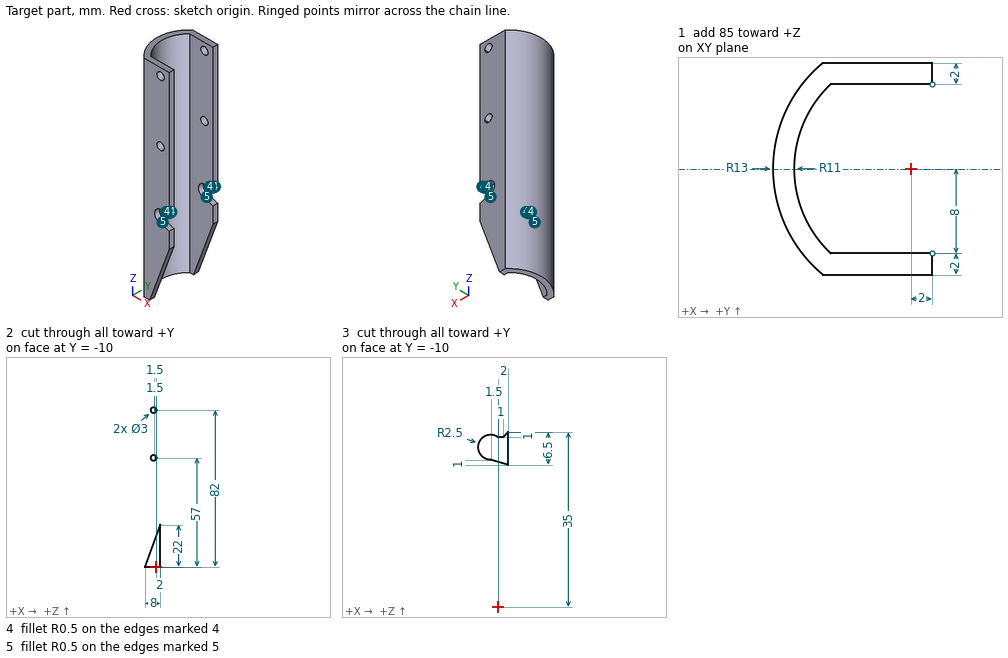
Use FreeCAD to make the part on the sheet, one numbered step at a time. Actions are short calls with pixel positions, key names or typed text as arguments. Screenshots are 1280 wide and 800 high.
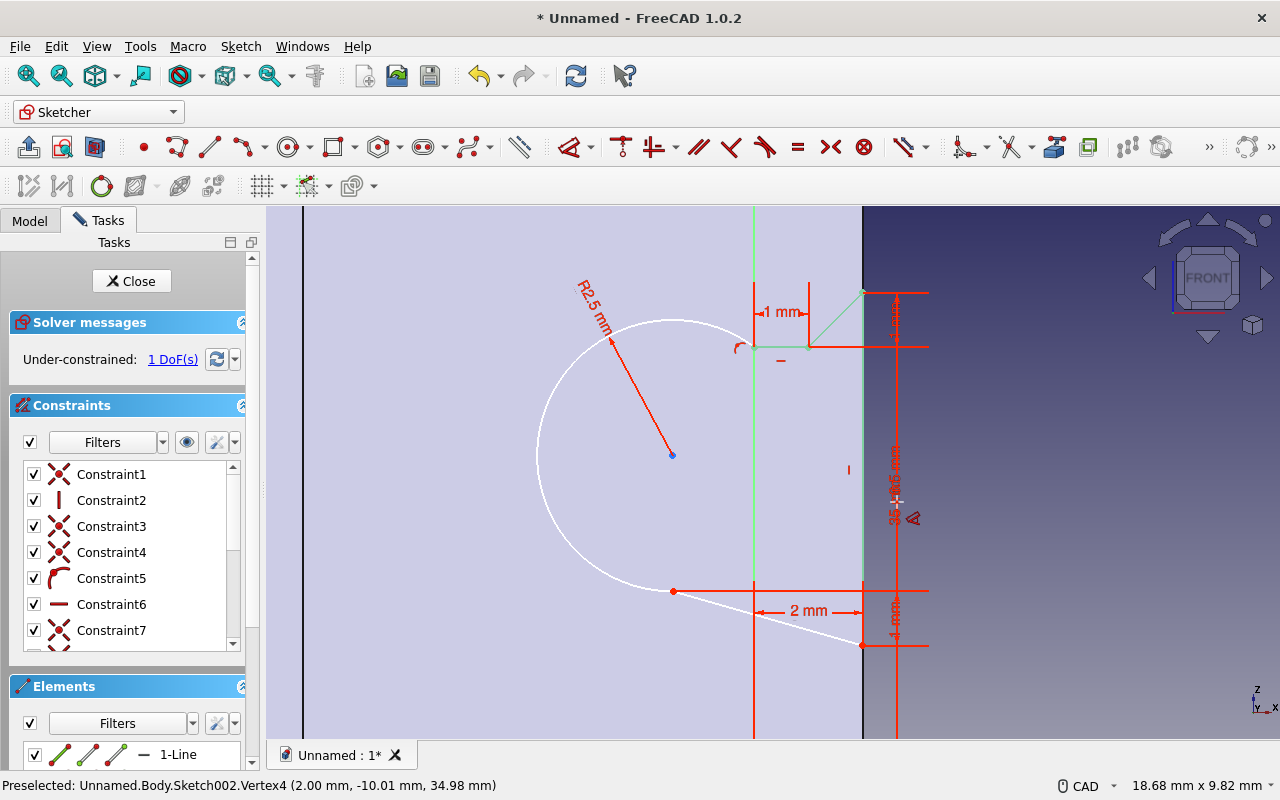
click(673, 591)
click(714, 557)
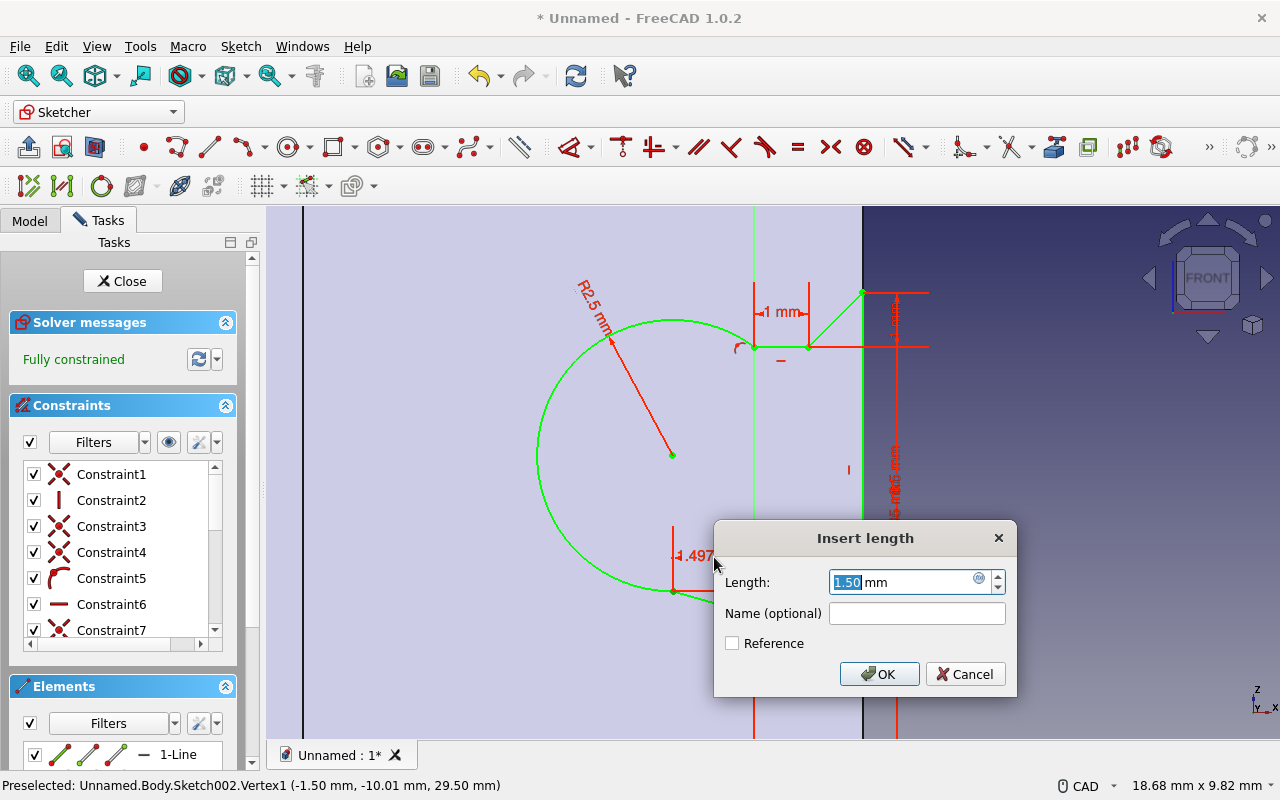
text(1.5)
key(Return)
key(Escape)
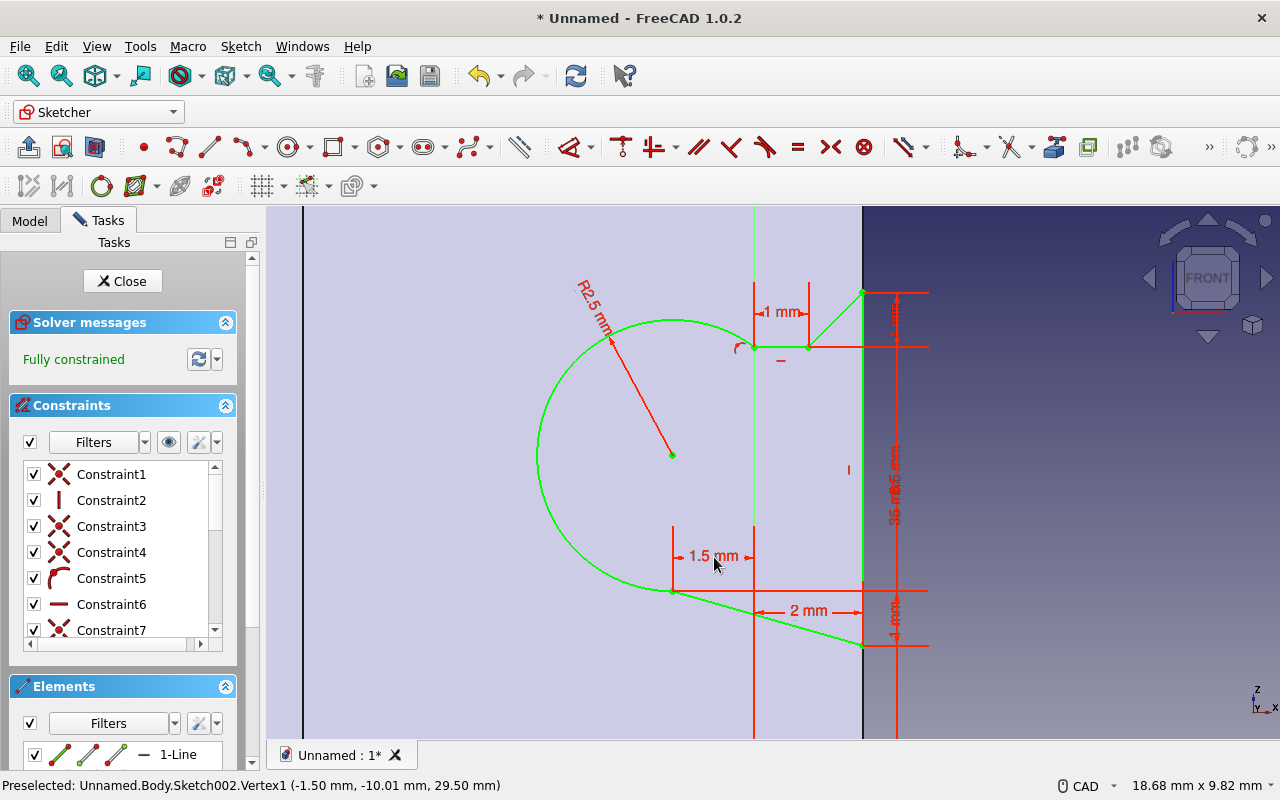
click(123, 281)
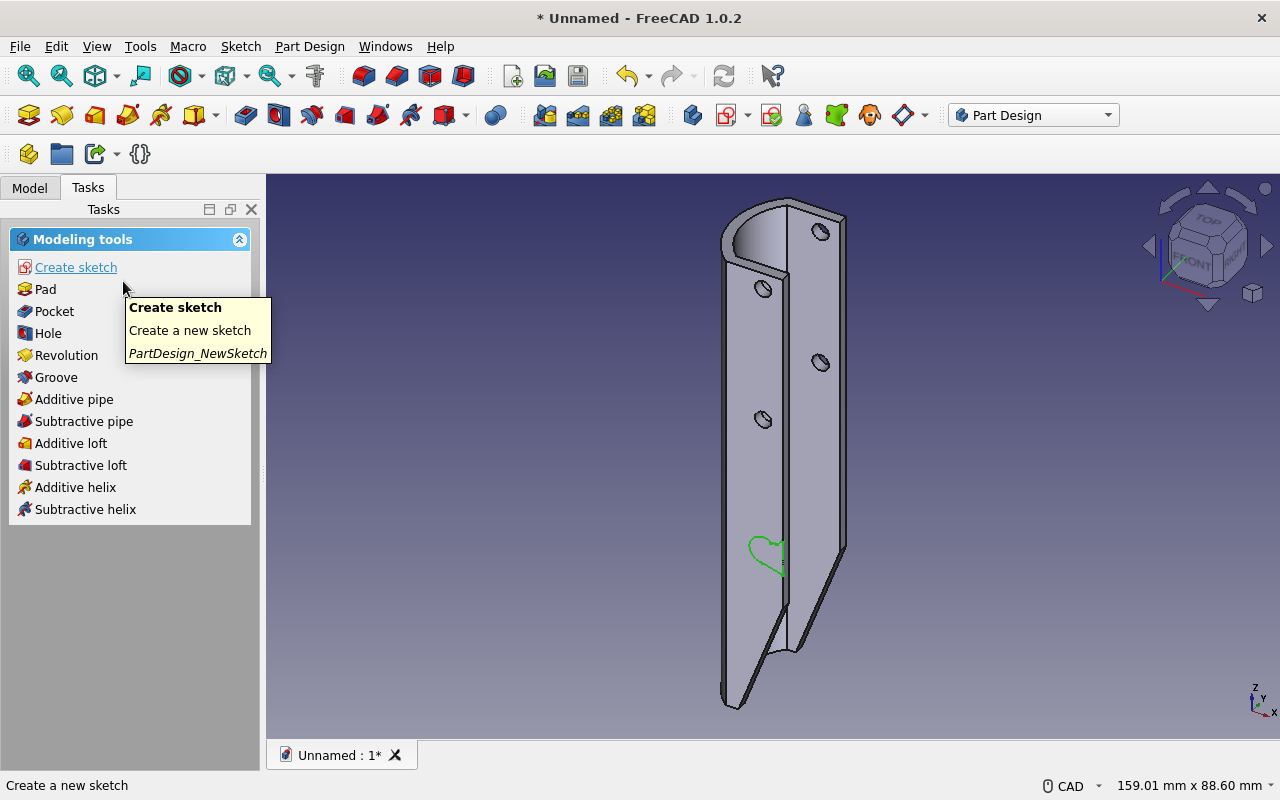
click(246, 116)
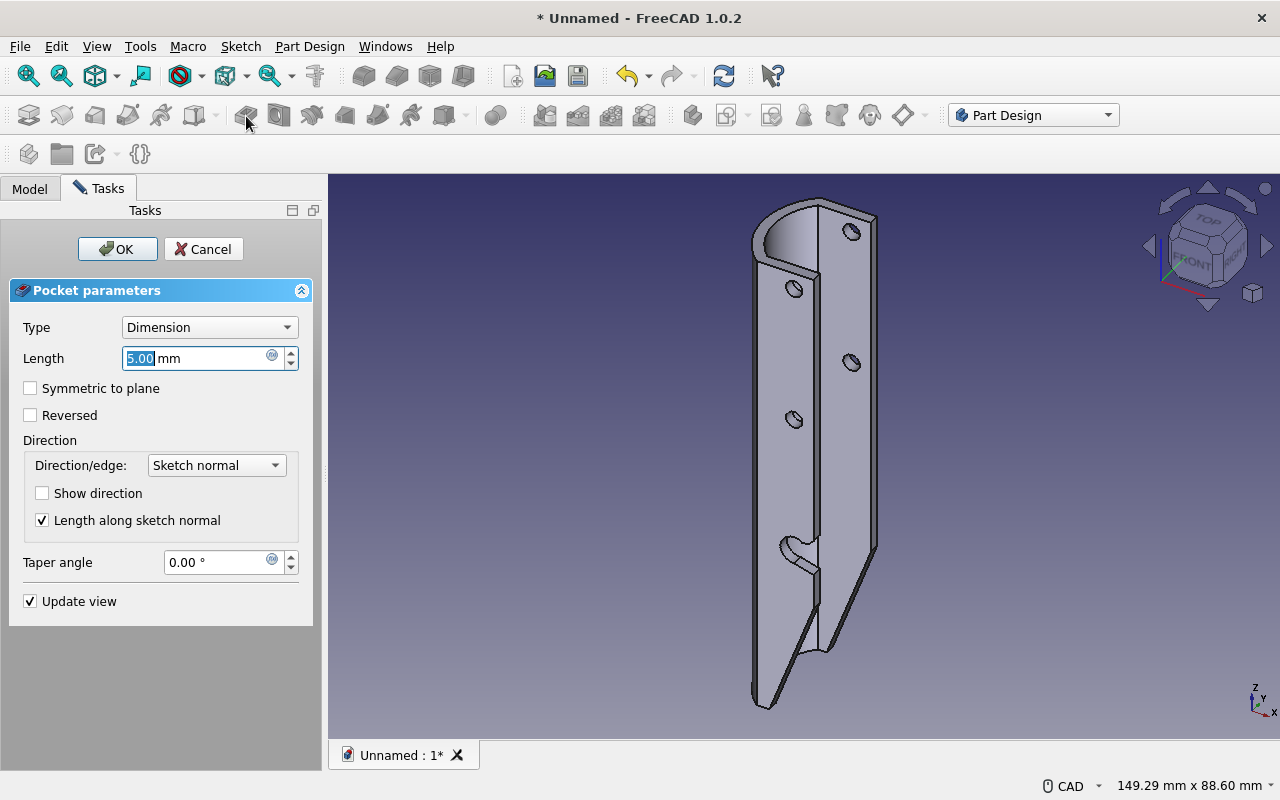
click(210, 328)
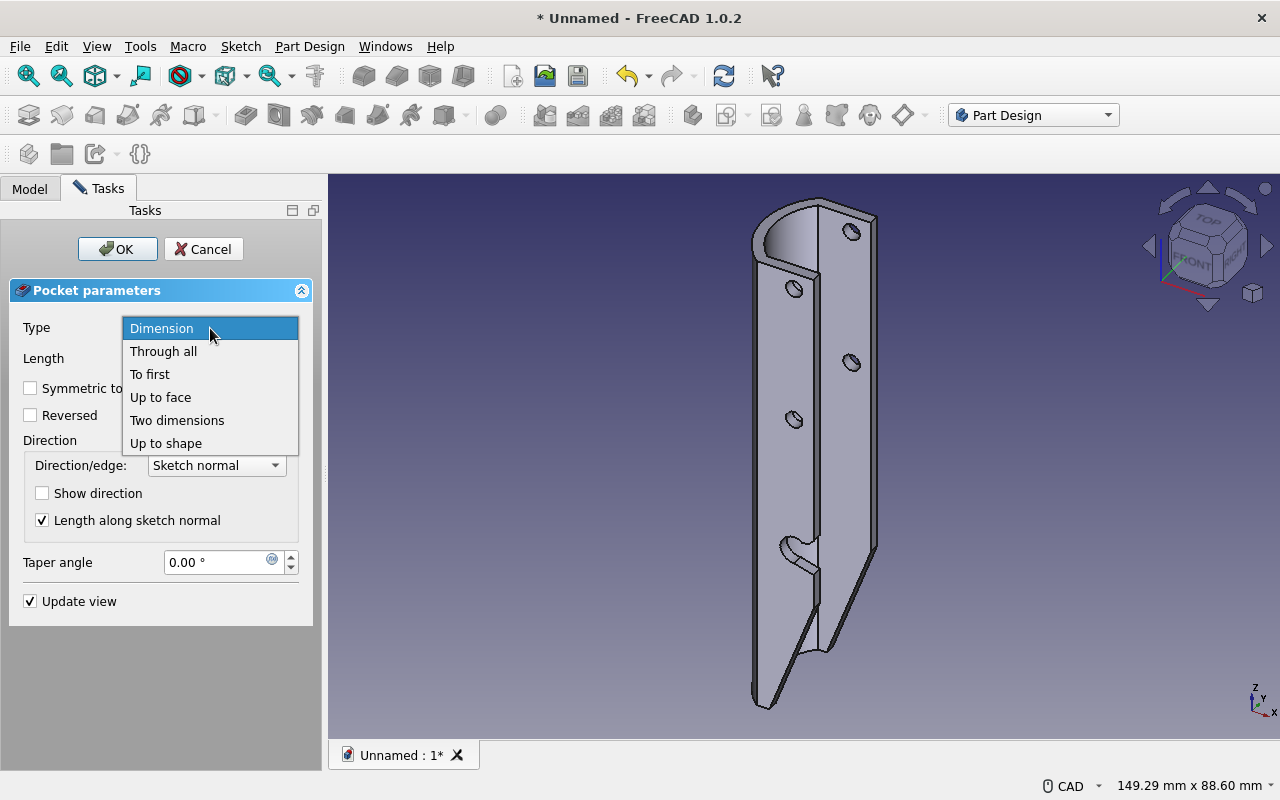
click(208, 352)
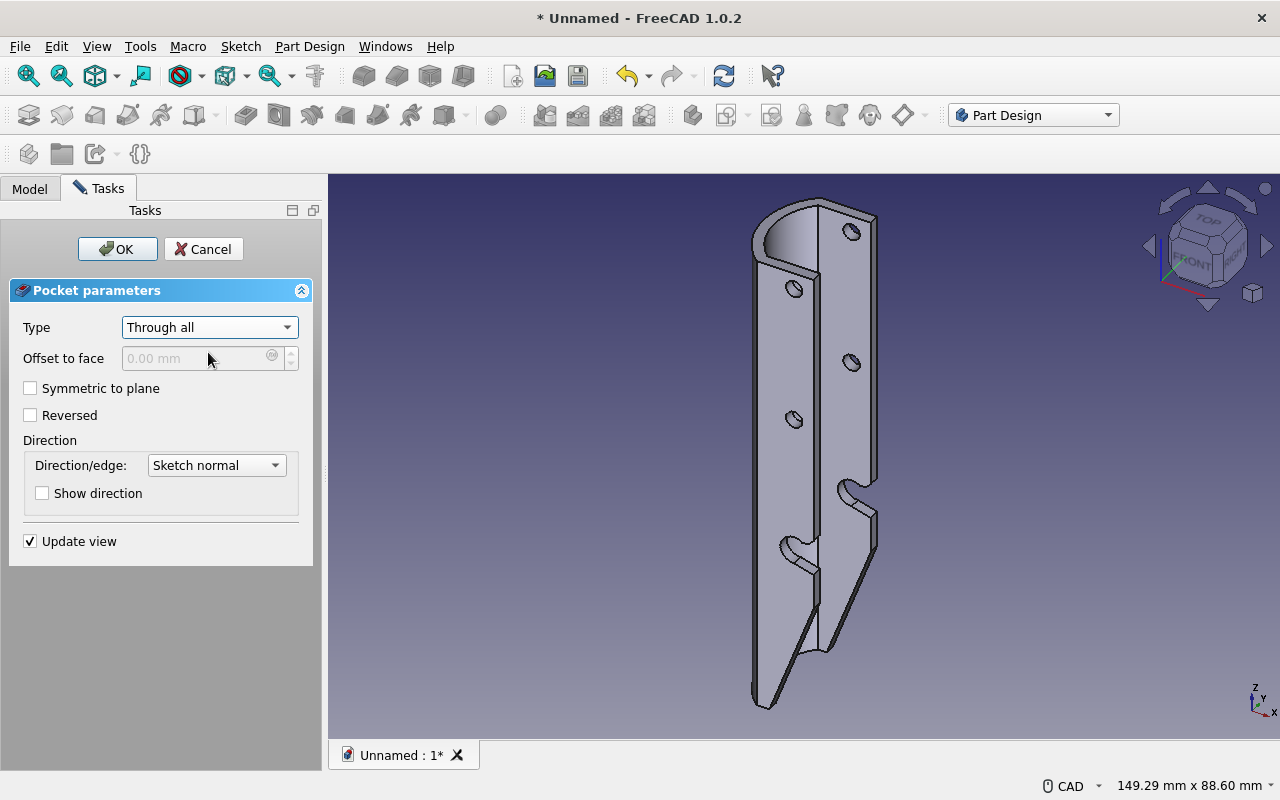
click(118, 249)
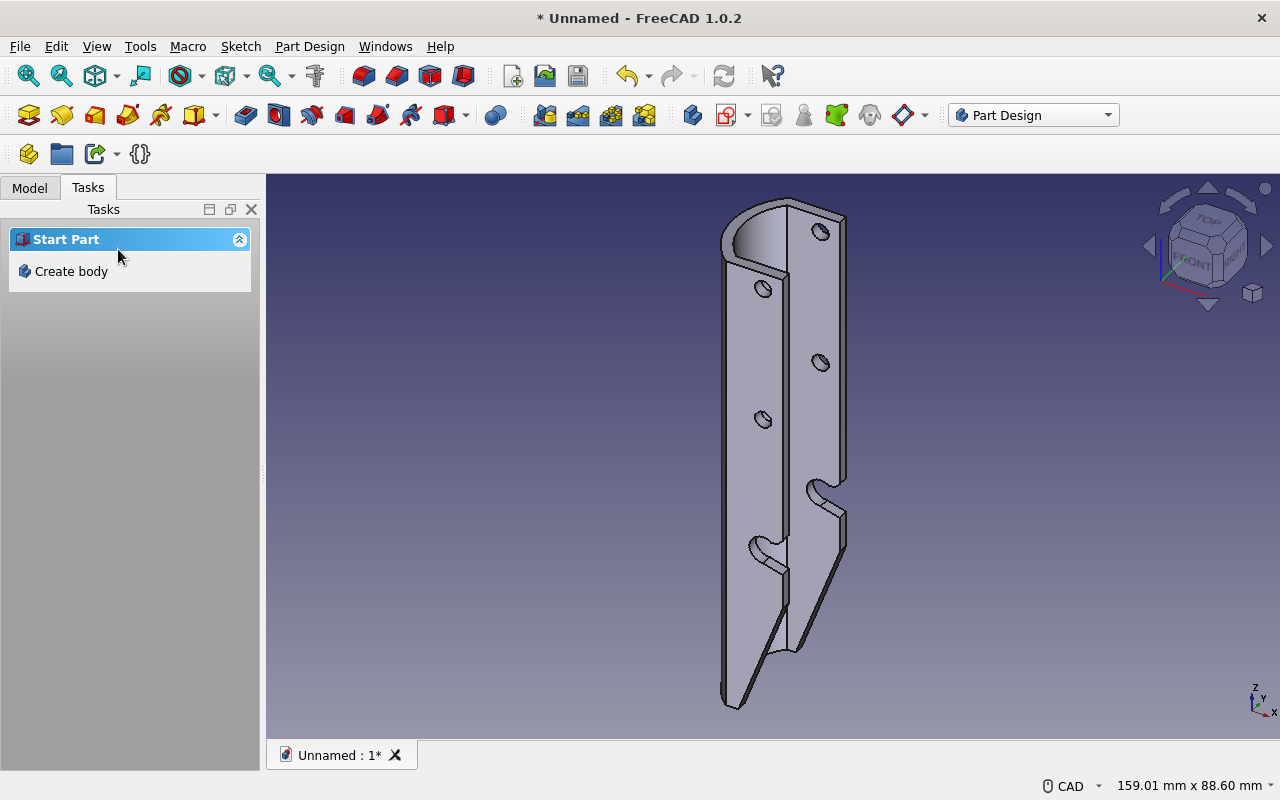
scroll(780, 540, up, 6)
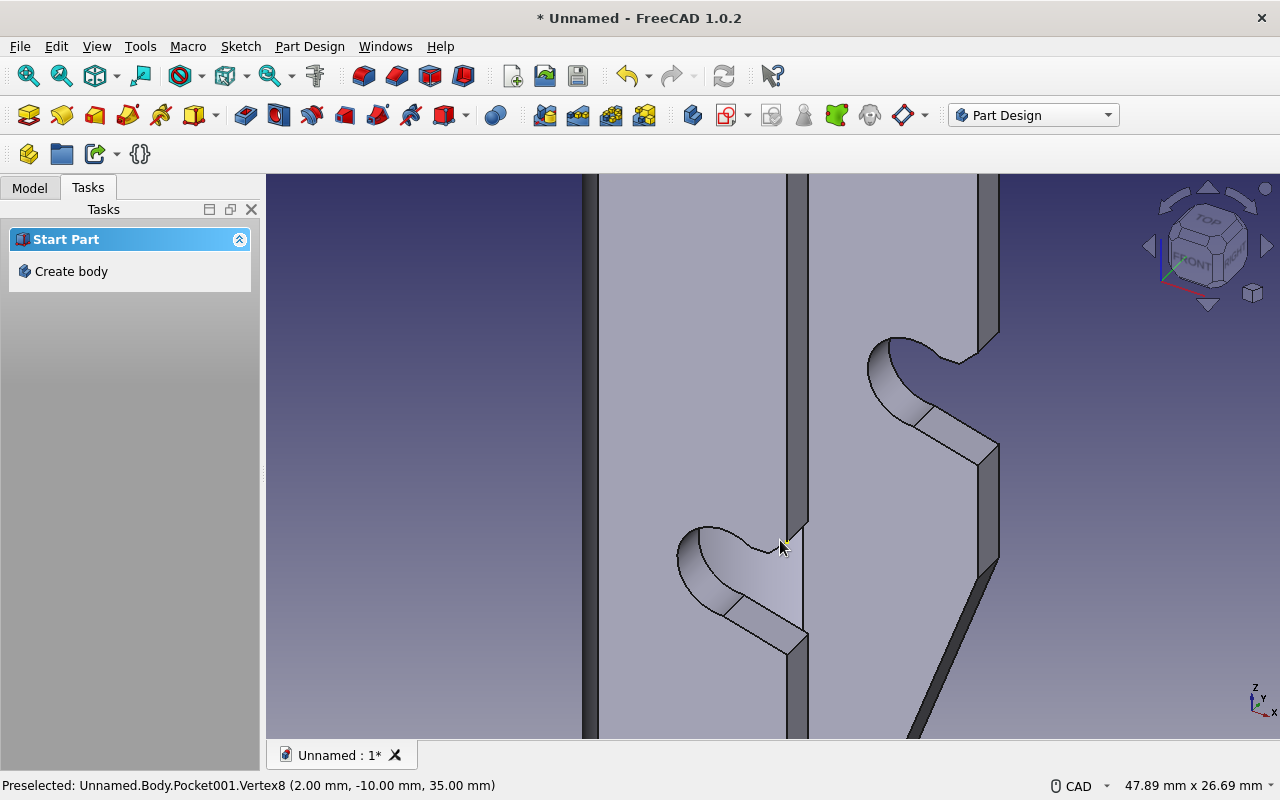
key(v)
key(f)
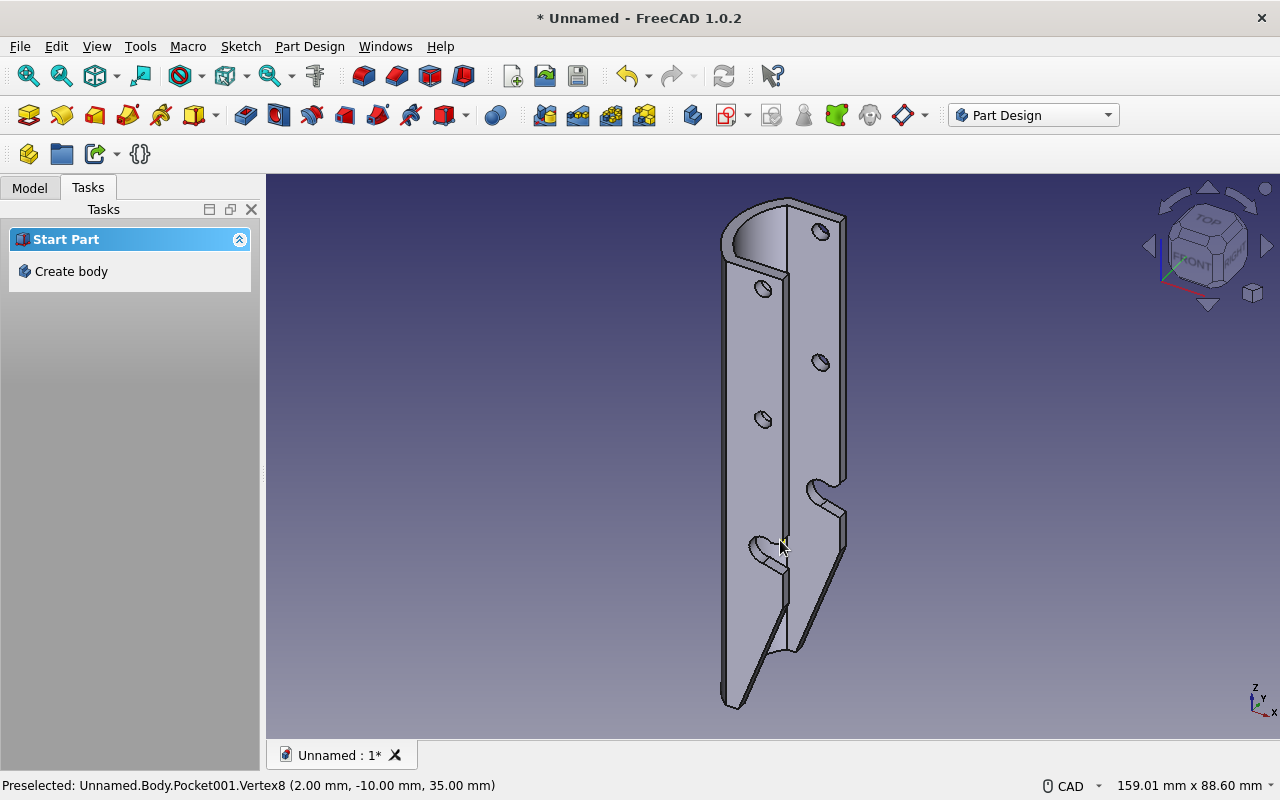
key(0)